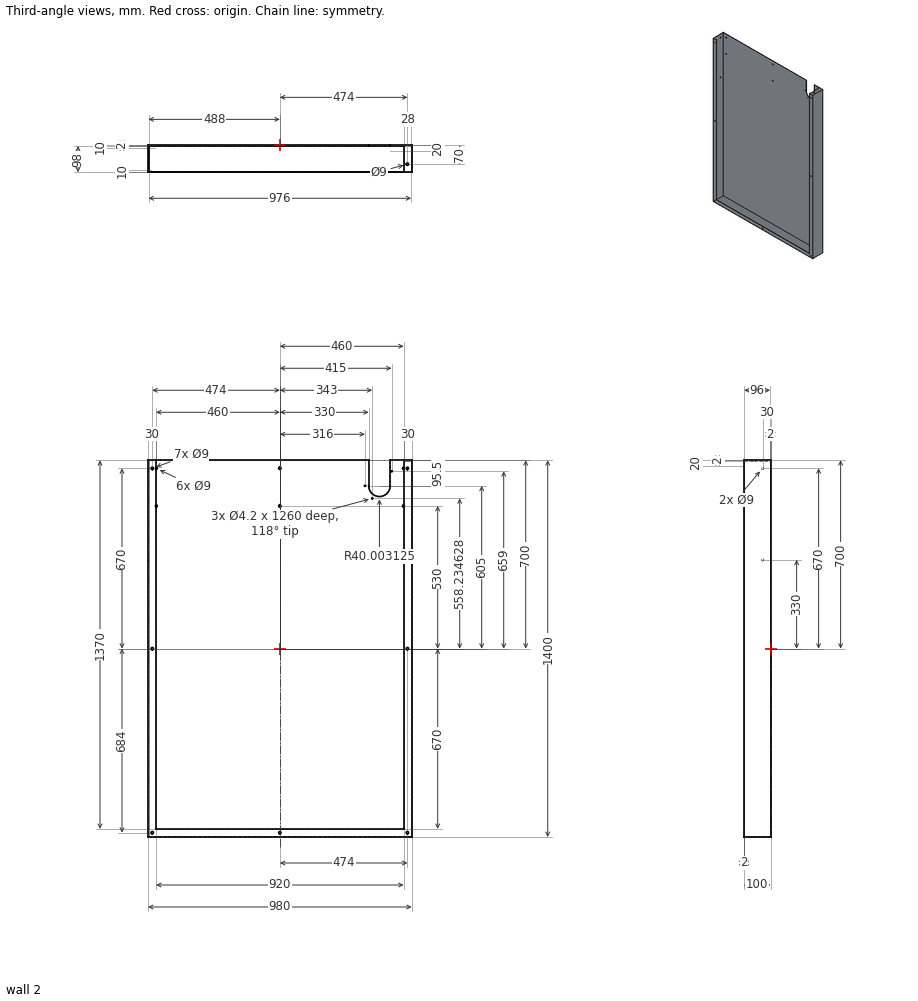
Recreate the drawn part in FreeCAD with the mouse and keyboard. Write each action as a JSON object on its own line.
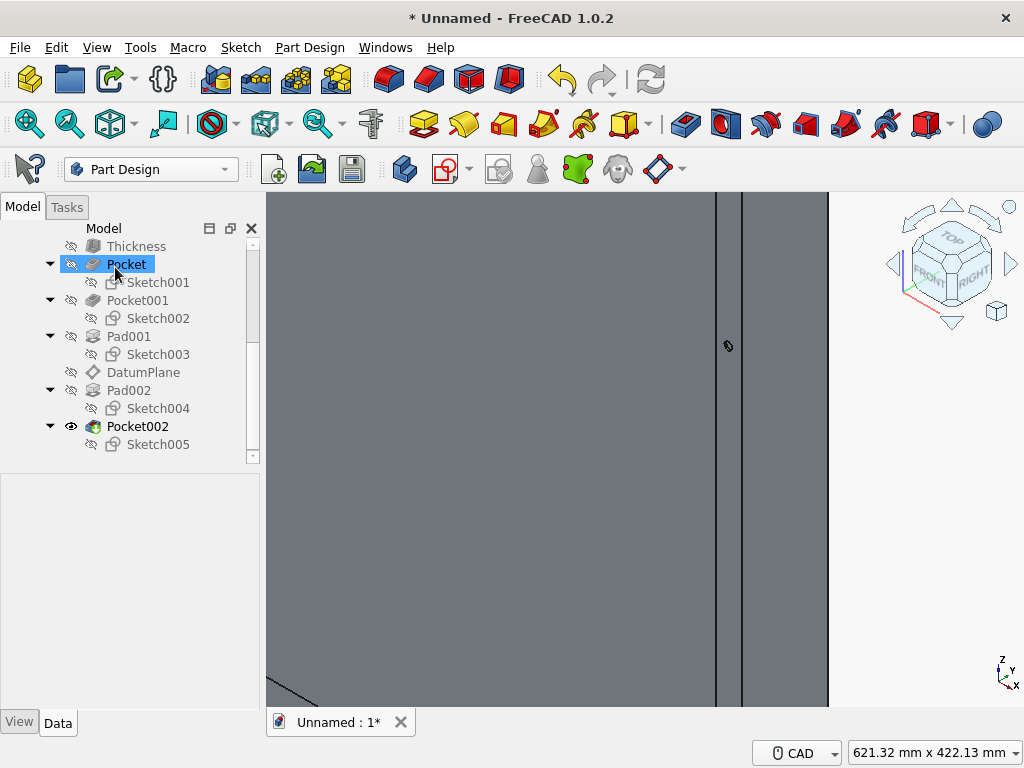
{"action": "left_click", "coordinate": [30, 124]}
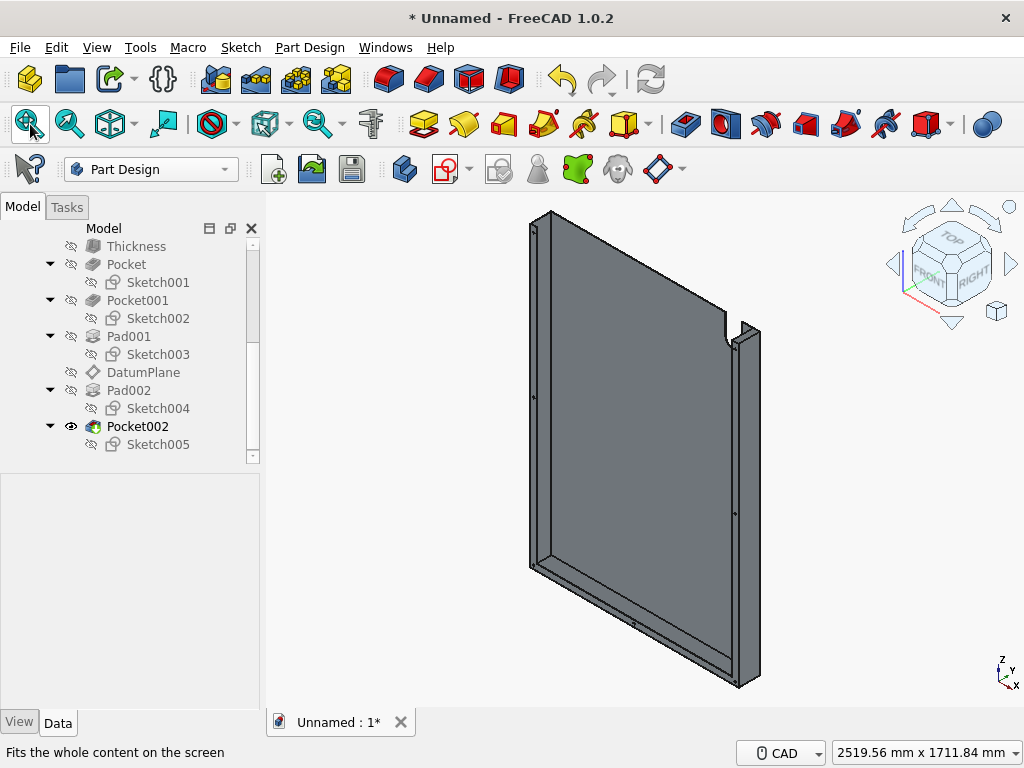
{"action": "scroll", "coordinate": [140, 350], "scroll_direction": "down", "scroll_amount": 3}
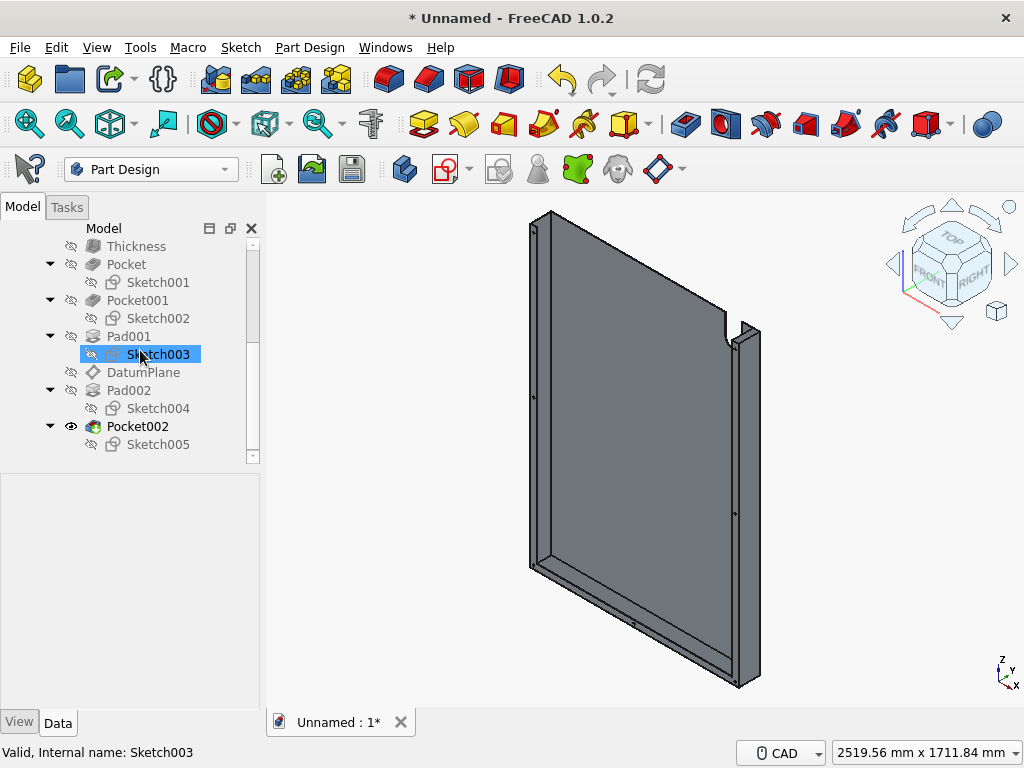
{"action": "scroll", "coordinate": [140, 350], "scroll_direction": "up", "scroll_amount": 15}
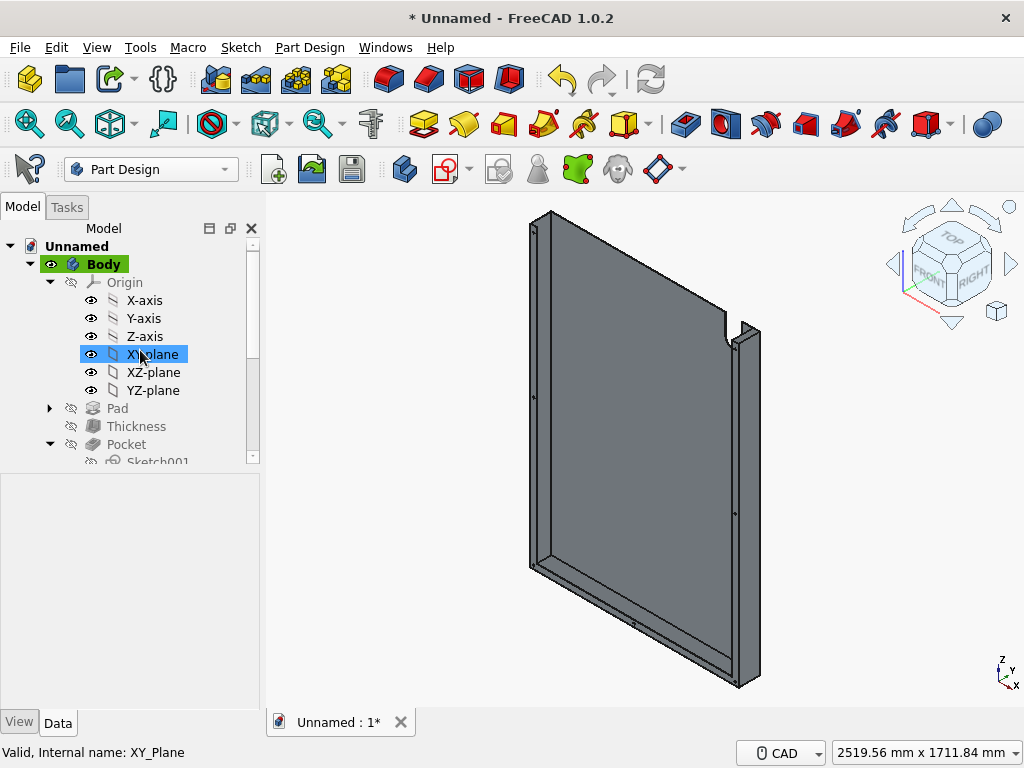
{"action": "left_click", "coordinate": [136, 354]}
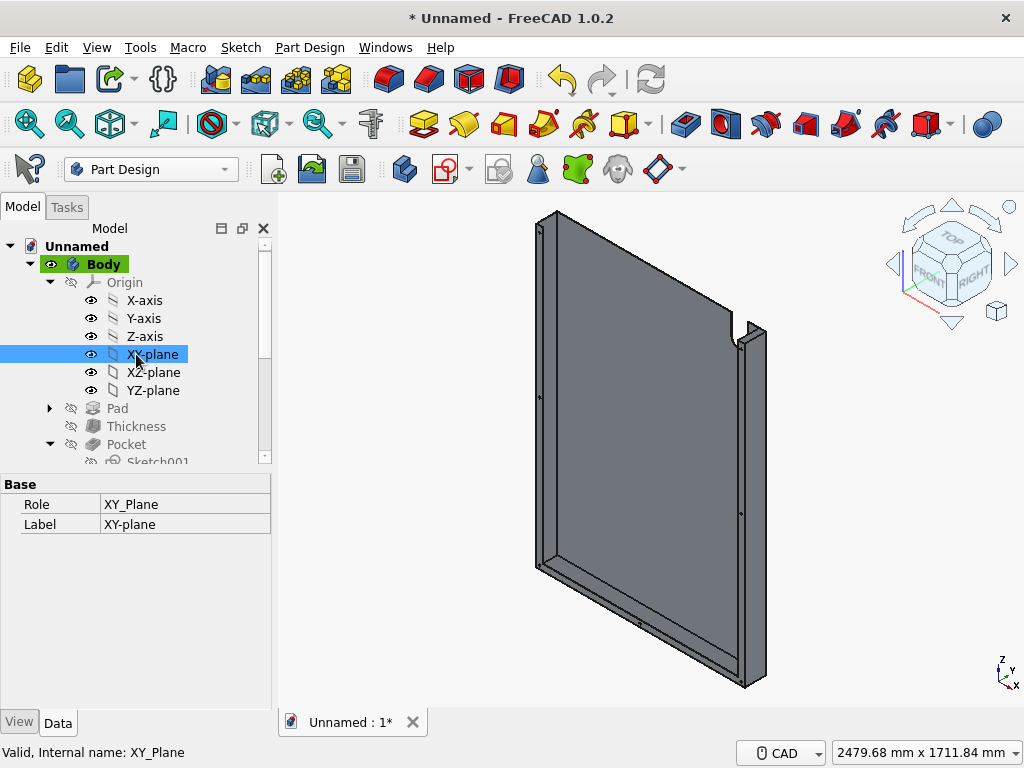
{"action": "left_click", "coordinate": [658, 170]}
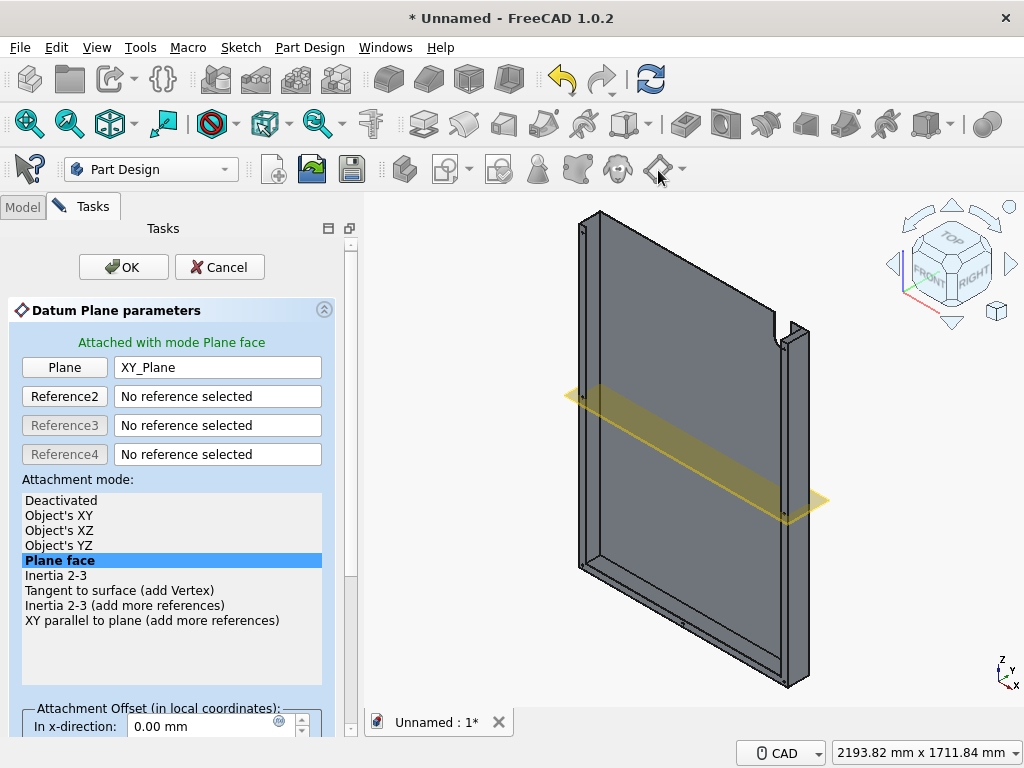
{"action": "scroll", "coordinate": [351, 487], "scroll_direction": "down", "scroll_amount": 3}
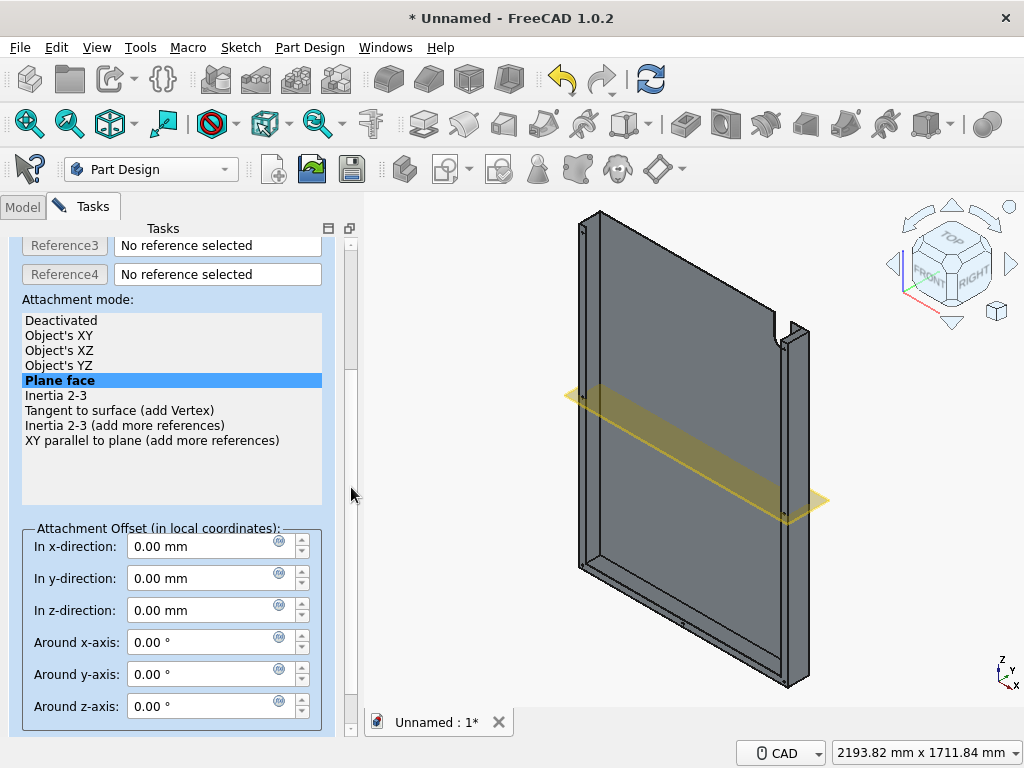
{"action": "triple_click", "coordinate": [210, 610]}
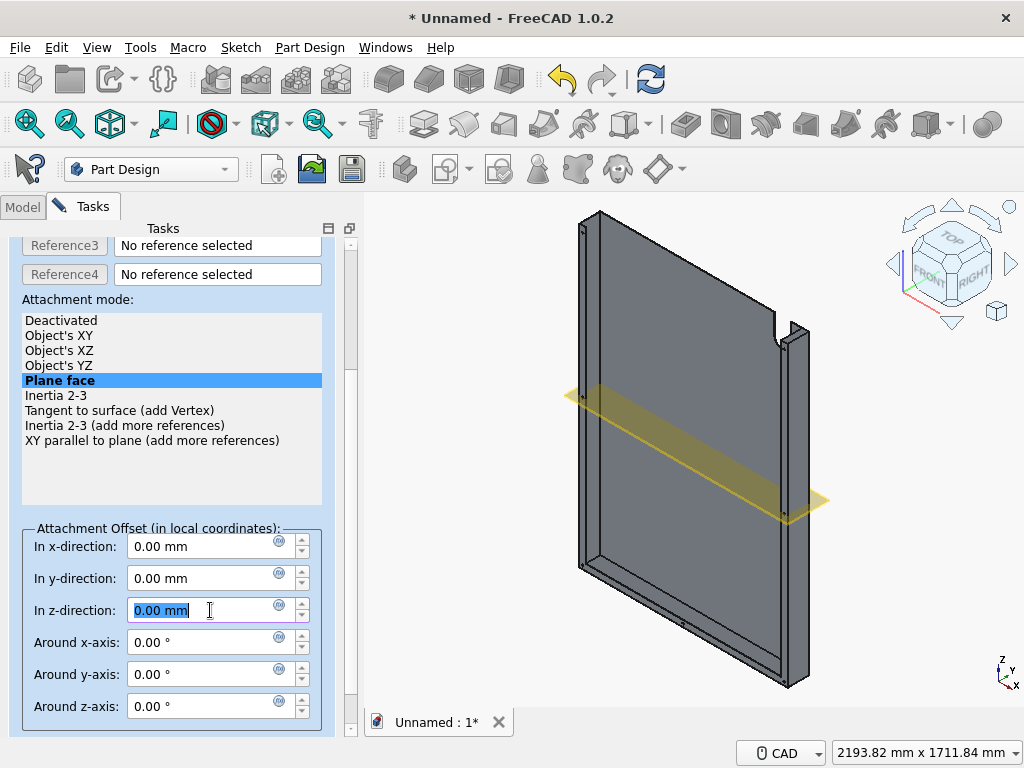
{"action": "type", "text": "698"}
{"action": "key", "text": "Tab"}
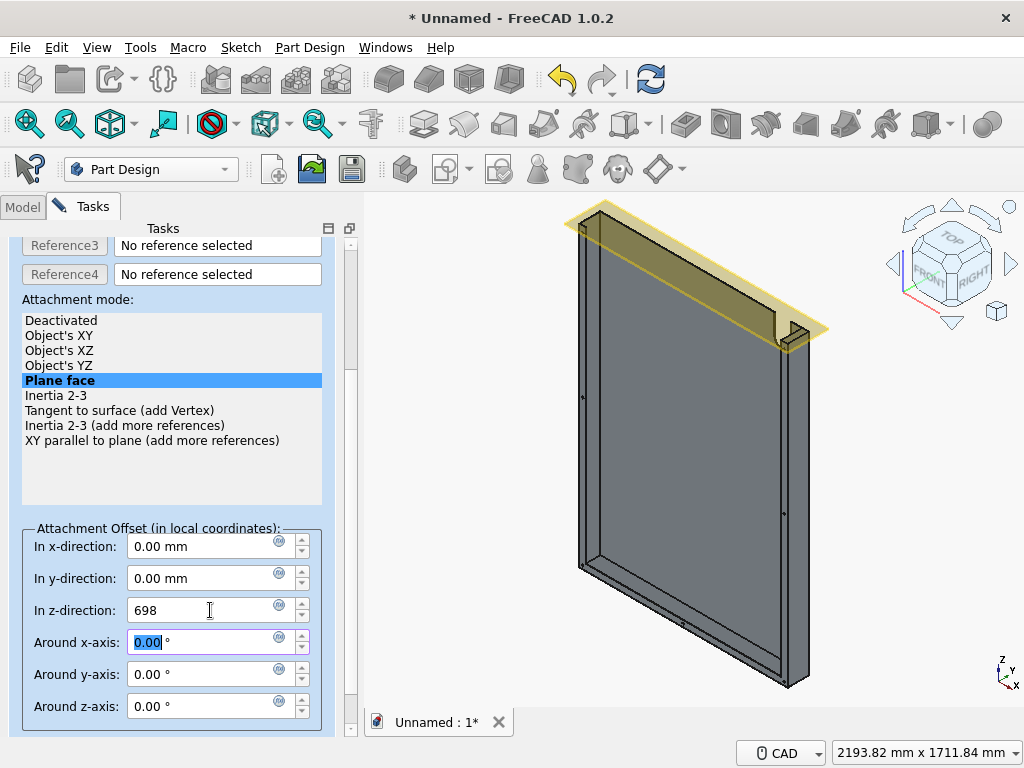
{"action": "scroll", "coordinate": [351, 487], "scroll_direction": "up", "scroll_amount": 4}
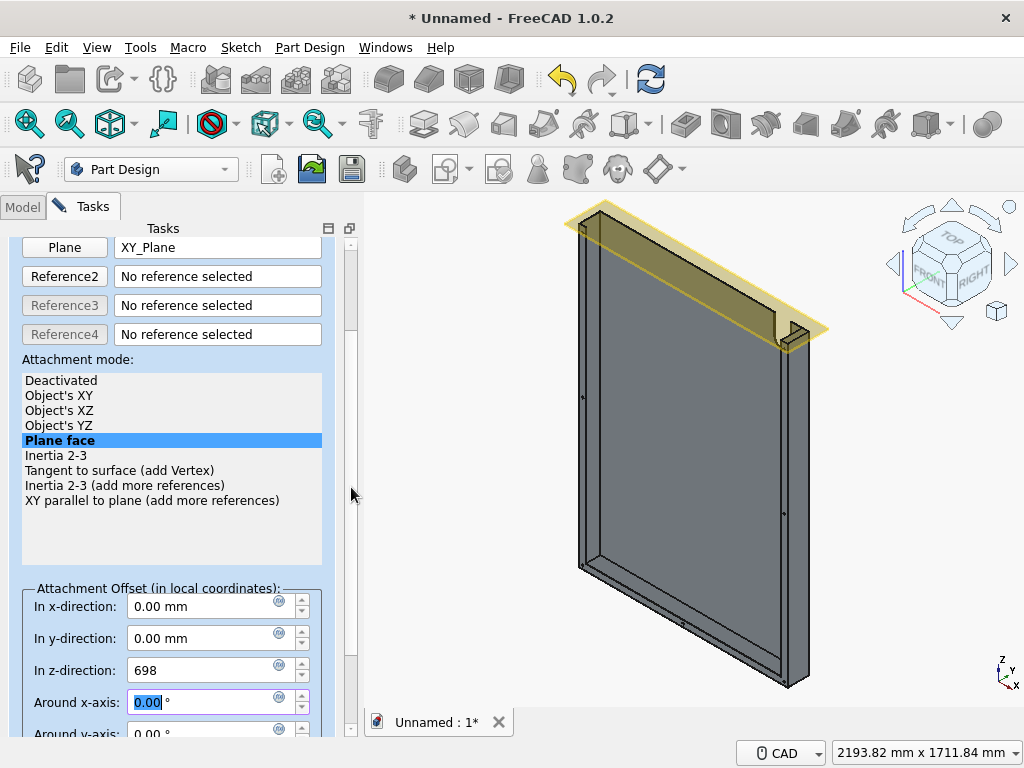
{"action": "left_click", "coordinate": [124, 267]}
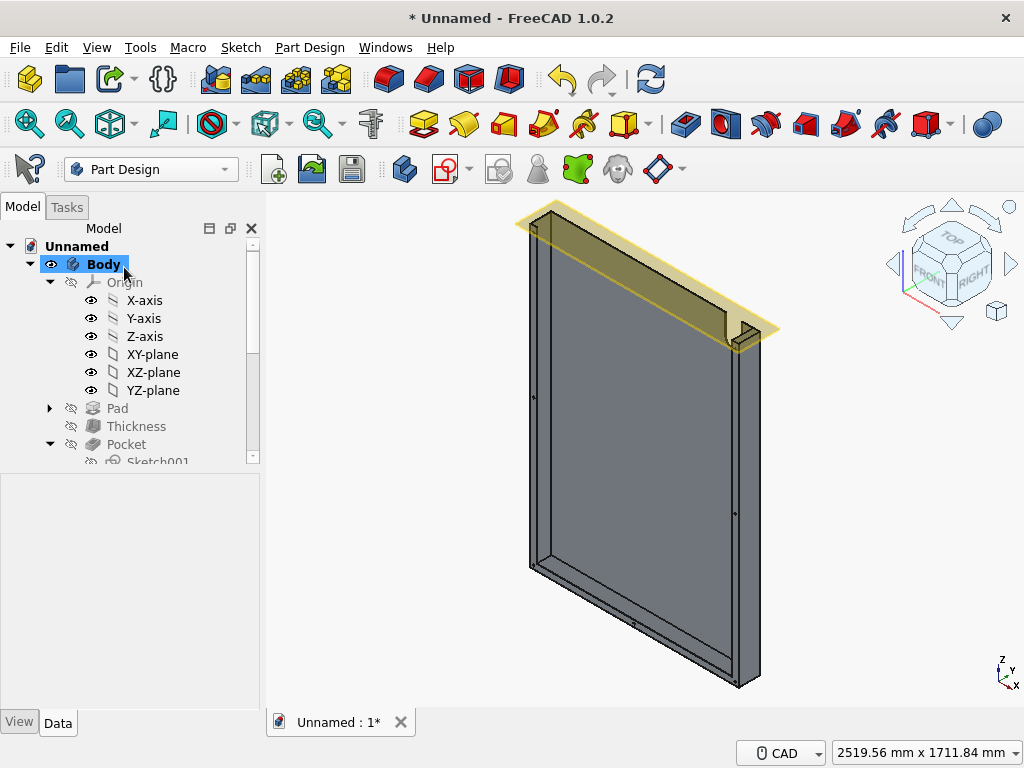
{"action": "scroll", "coordinate": [100, 350], "scroll_direction": "down", "scroll_amount": 3}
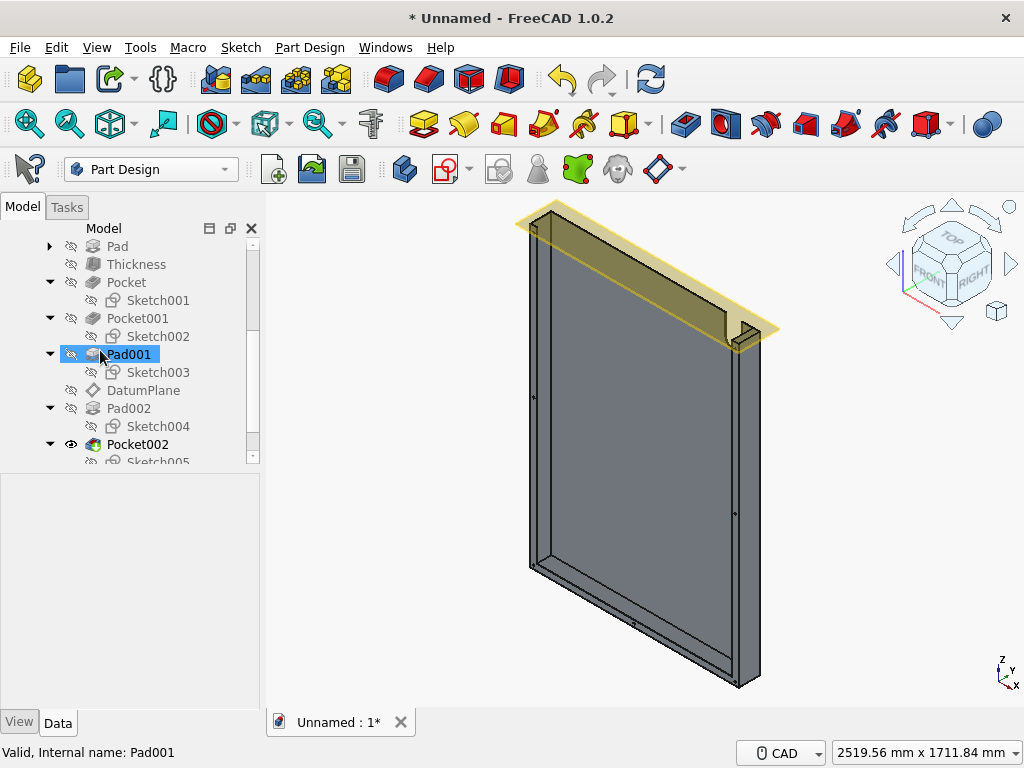
{"action": "scroll", "coordinate": [140, 350], "scroll_direction": "up", "scroll_amount": 15}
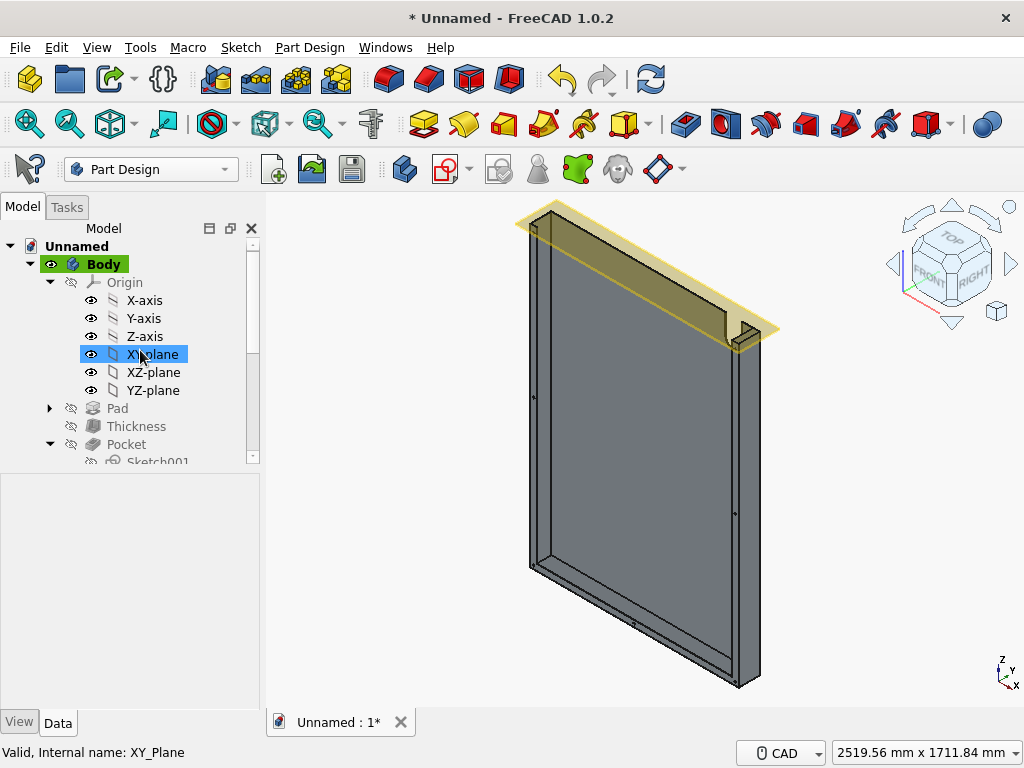
{"action": "scroll", "coordinate": [100, 350], "scroll_direction": "down", "scroll_amount": 6}